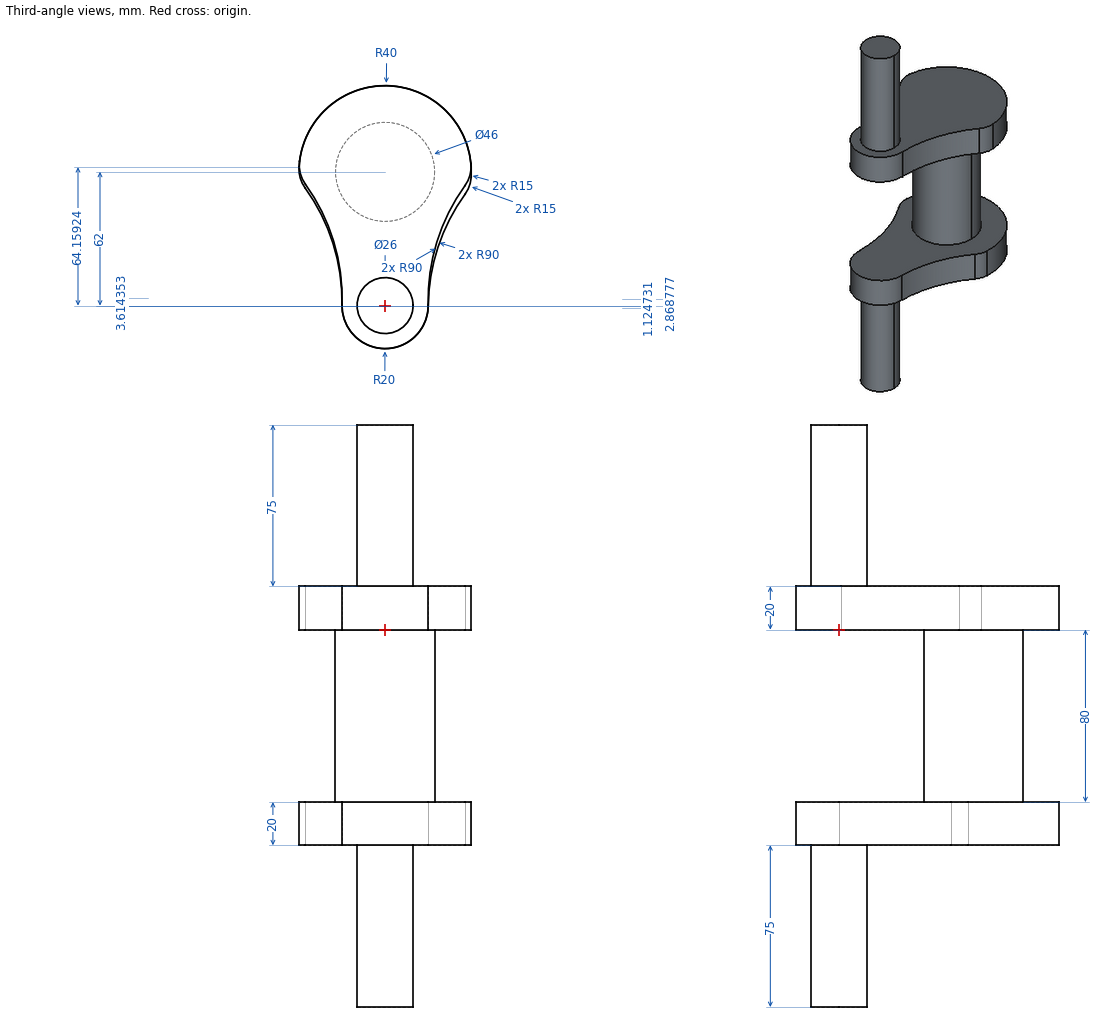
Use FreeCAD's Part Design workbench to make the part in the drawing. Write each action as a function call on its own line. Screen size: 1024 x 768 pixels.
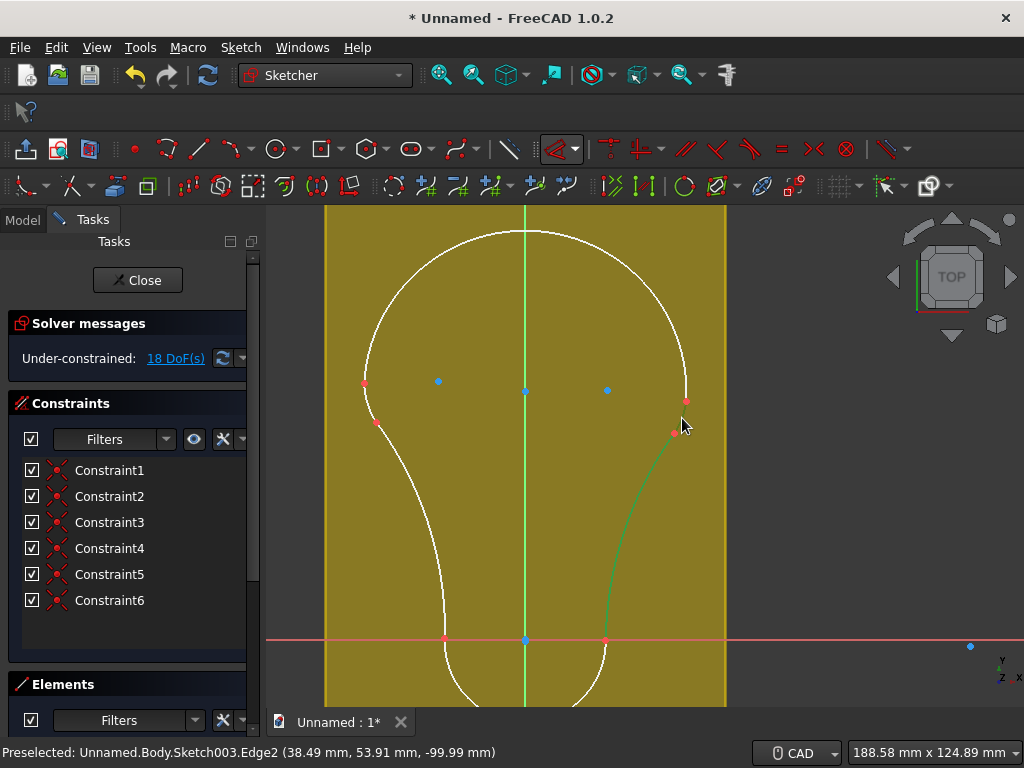
click(750, 150)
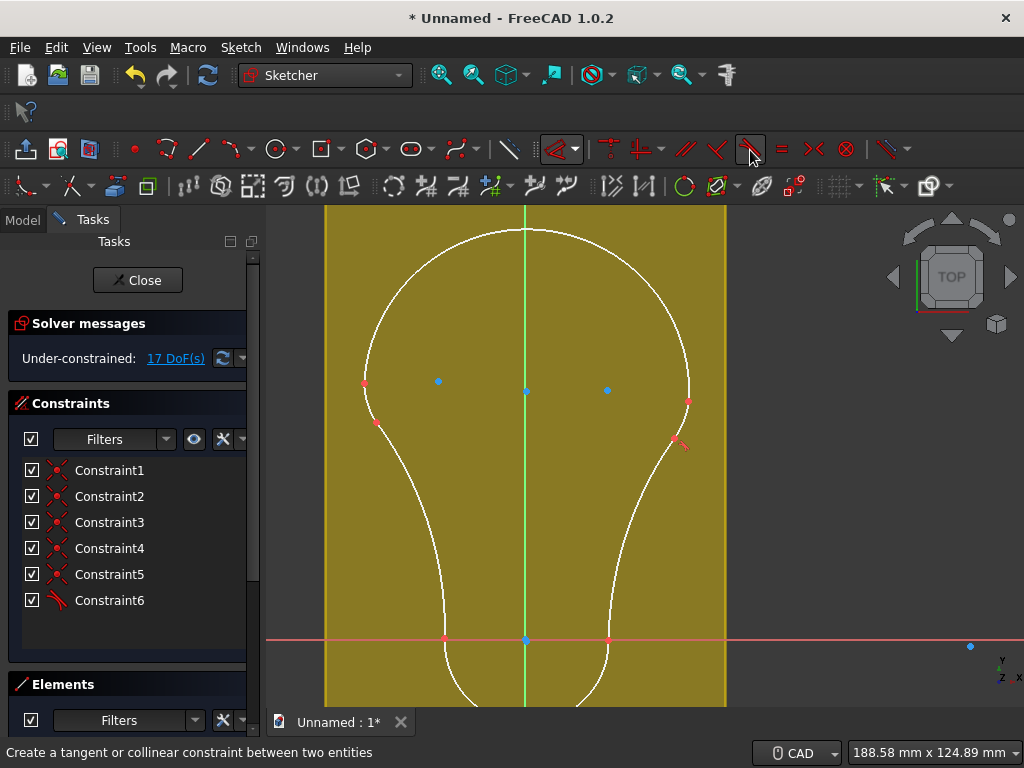
click(642, 494)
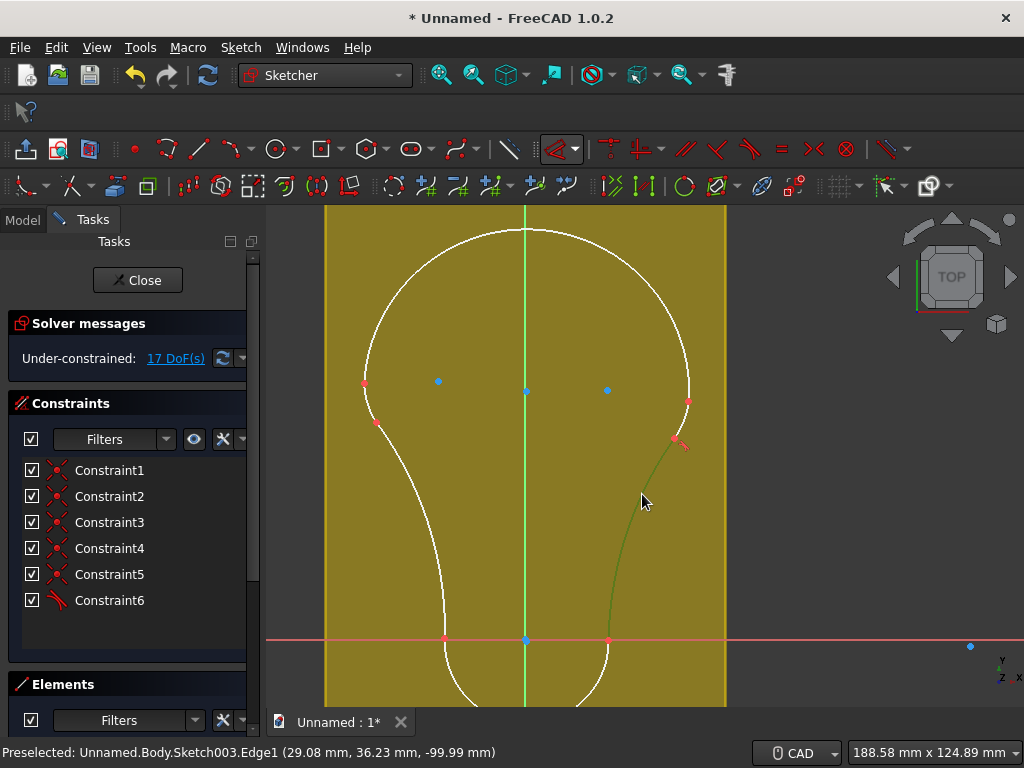
scroll(681, 417, down, 2)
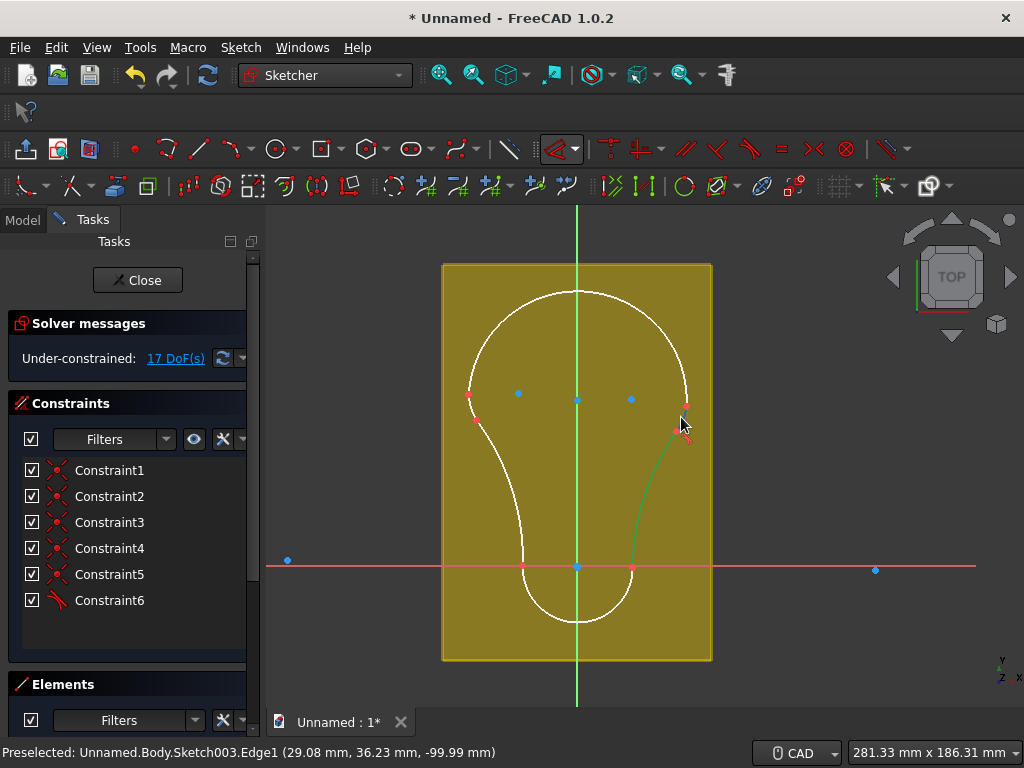
click(545, 611)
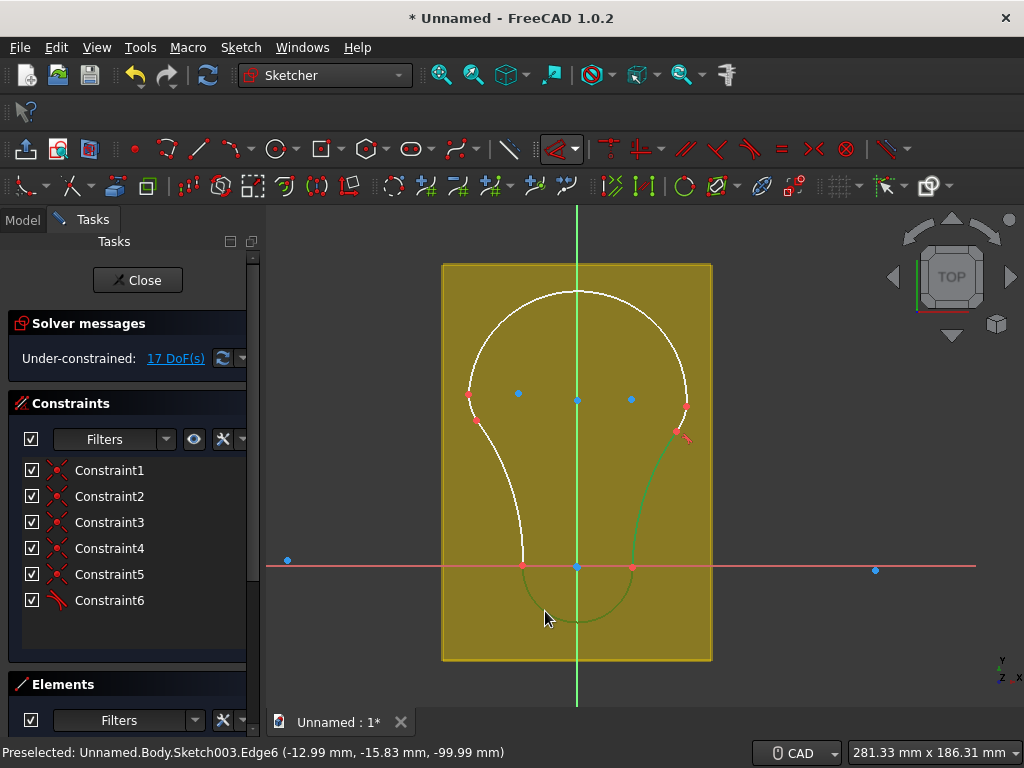
click(750, 150)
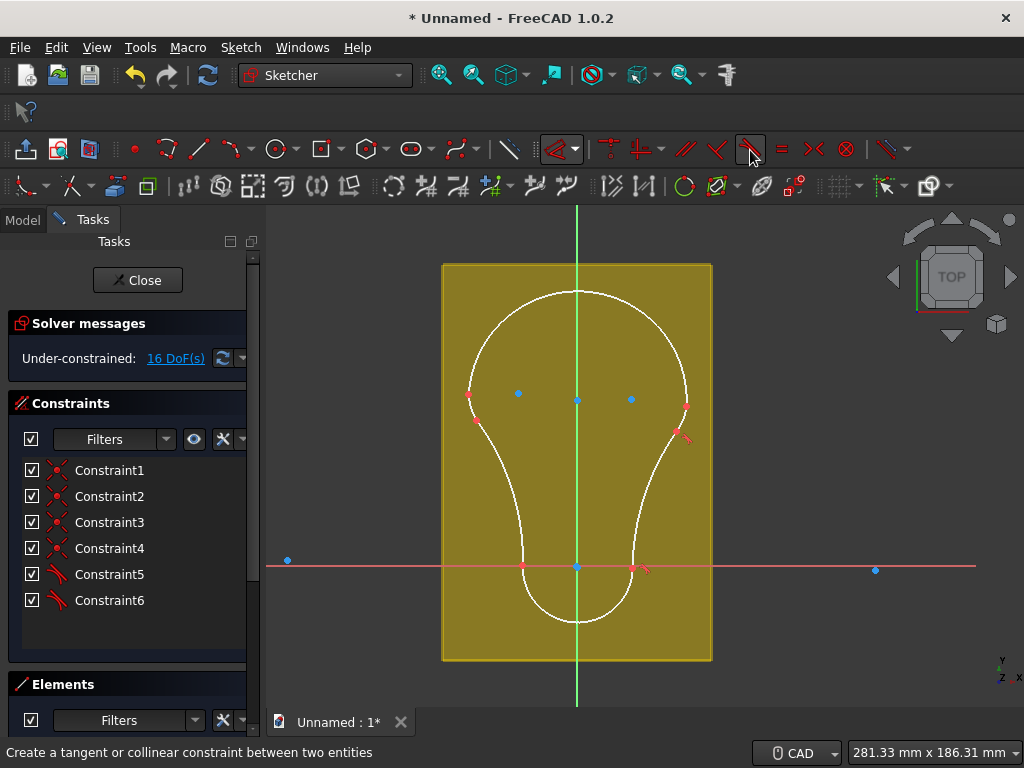
click(683, 420)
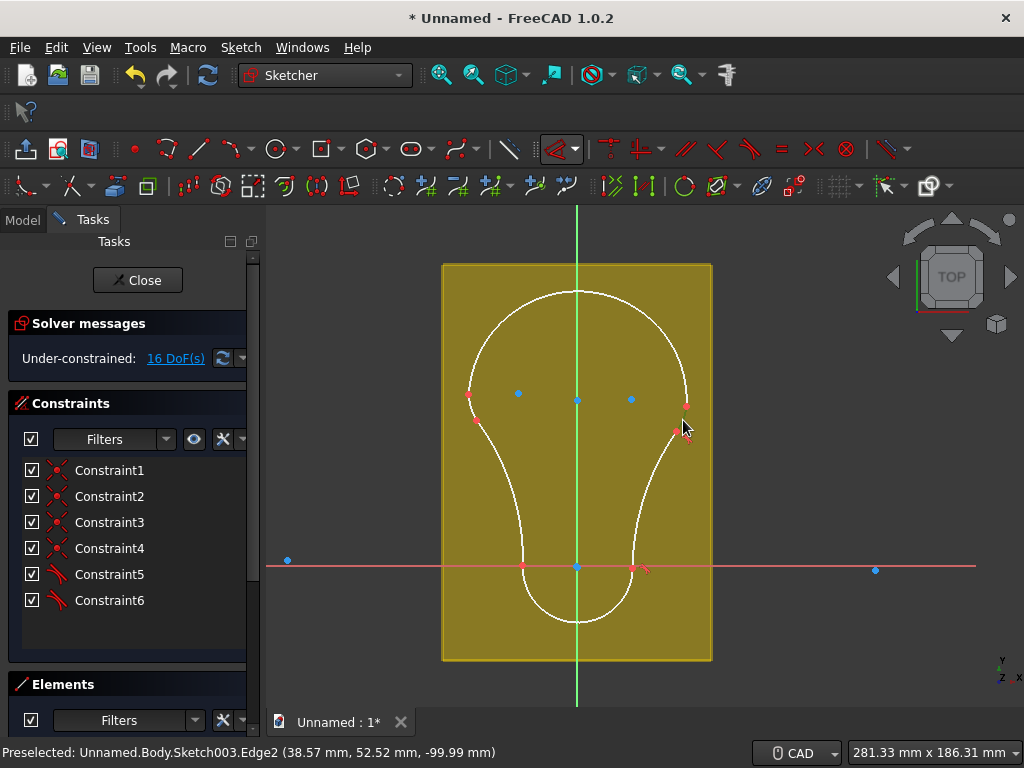
click(647, 316)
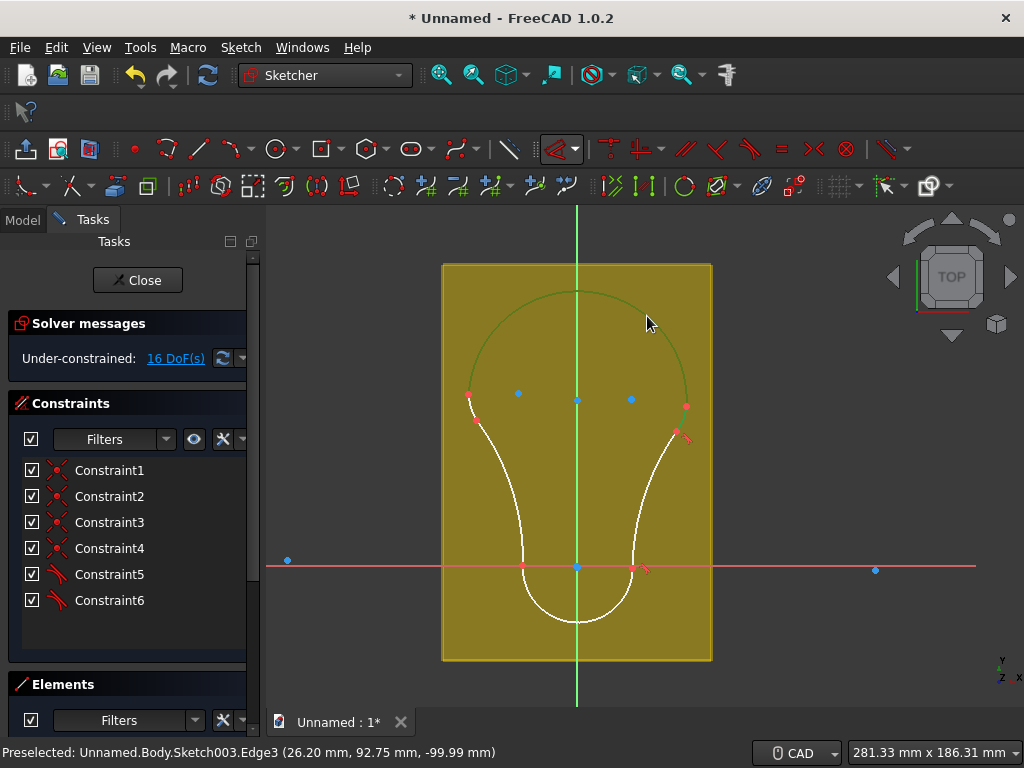
click(750, 150)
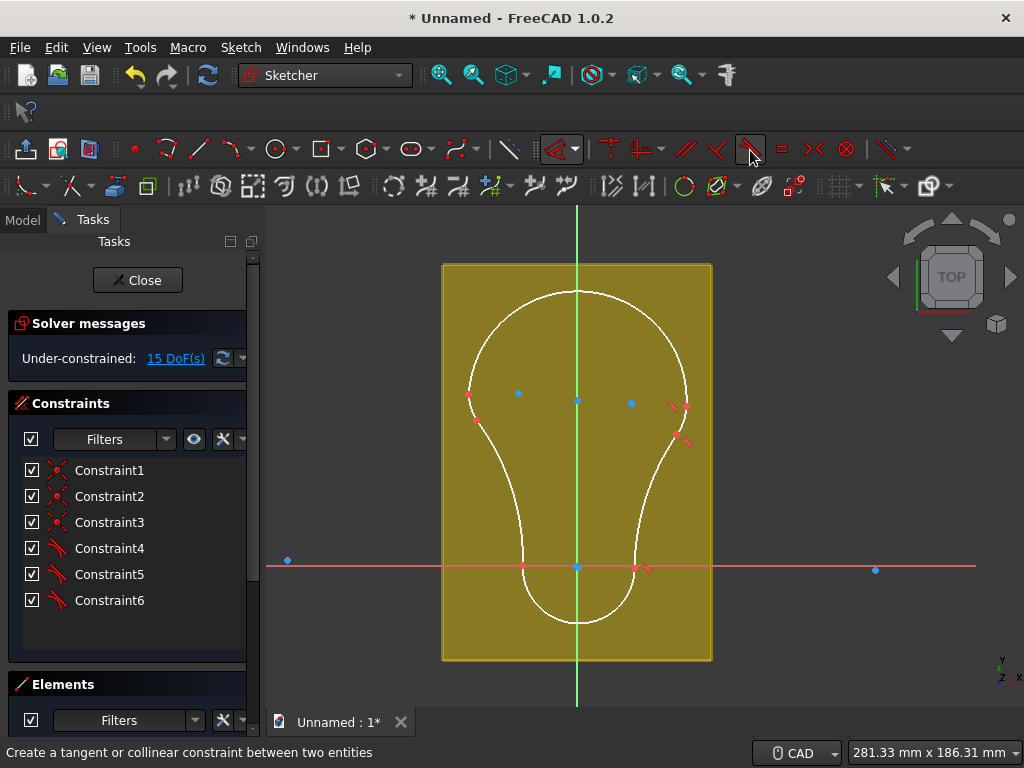
click(647, 316)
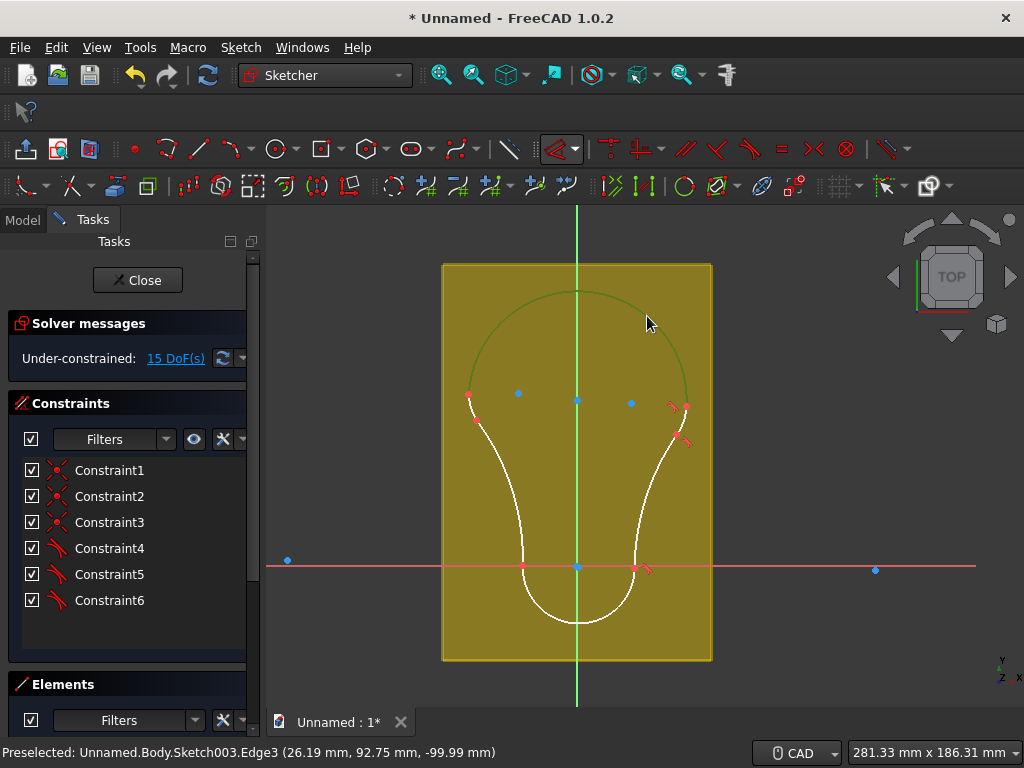
click(471, 408)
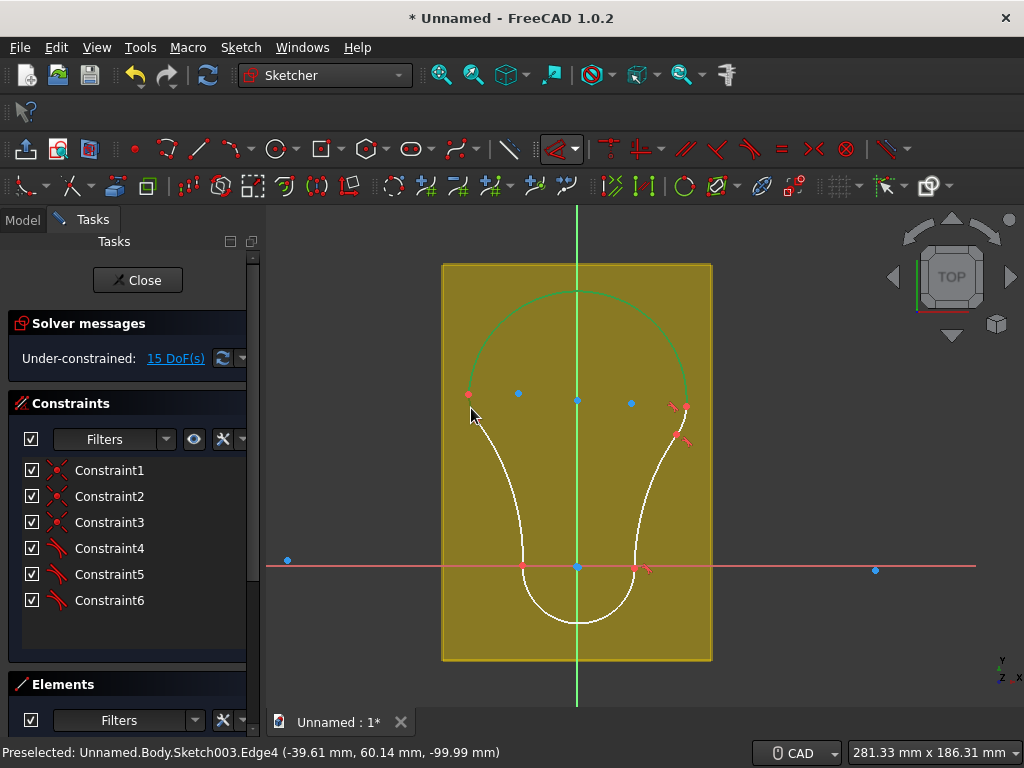
key(t)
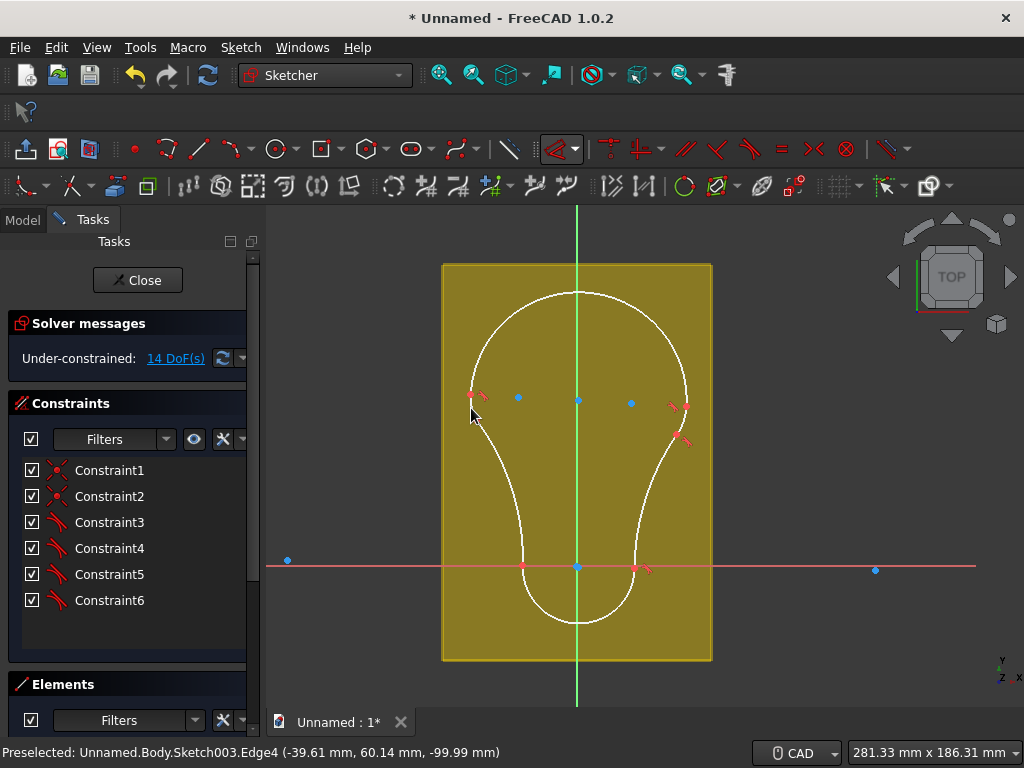
click(472, 408)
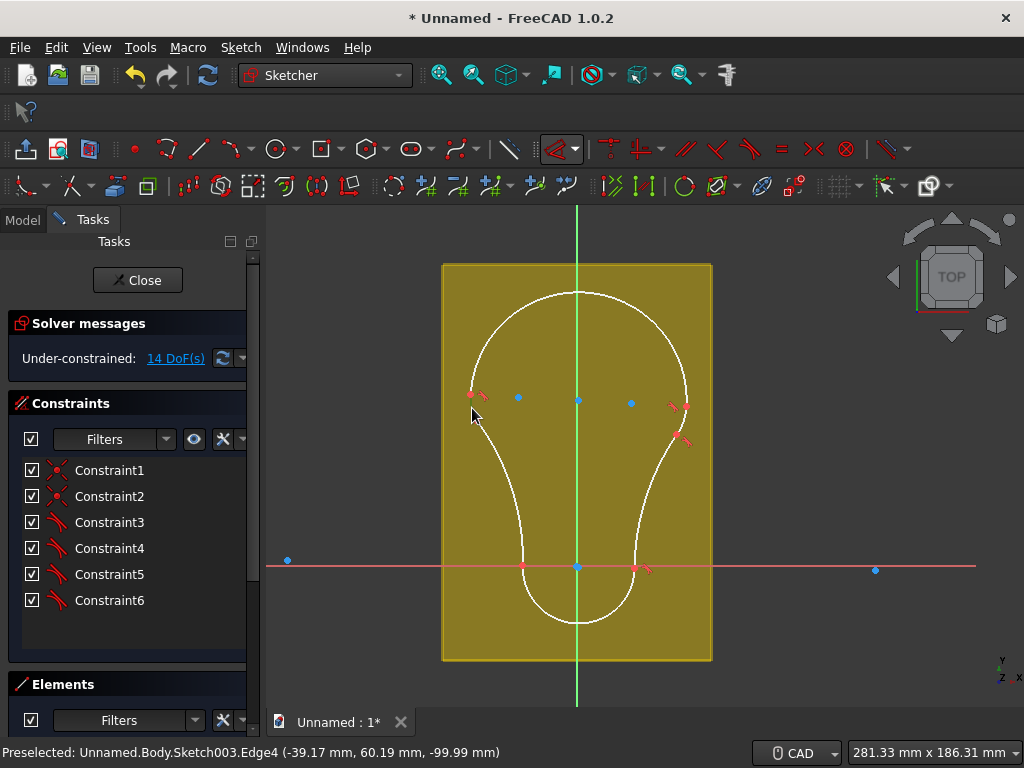
click(519, 519)